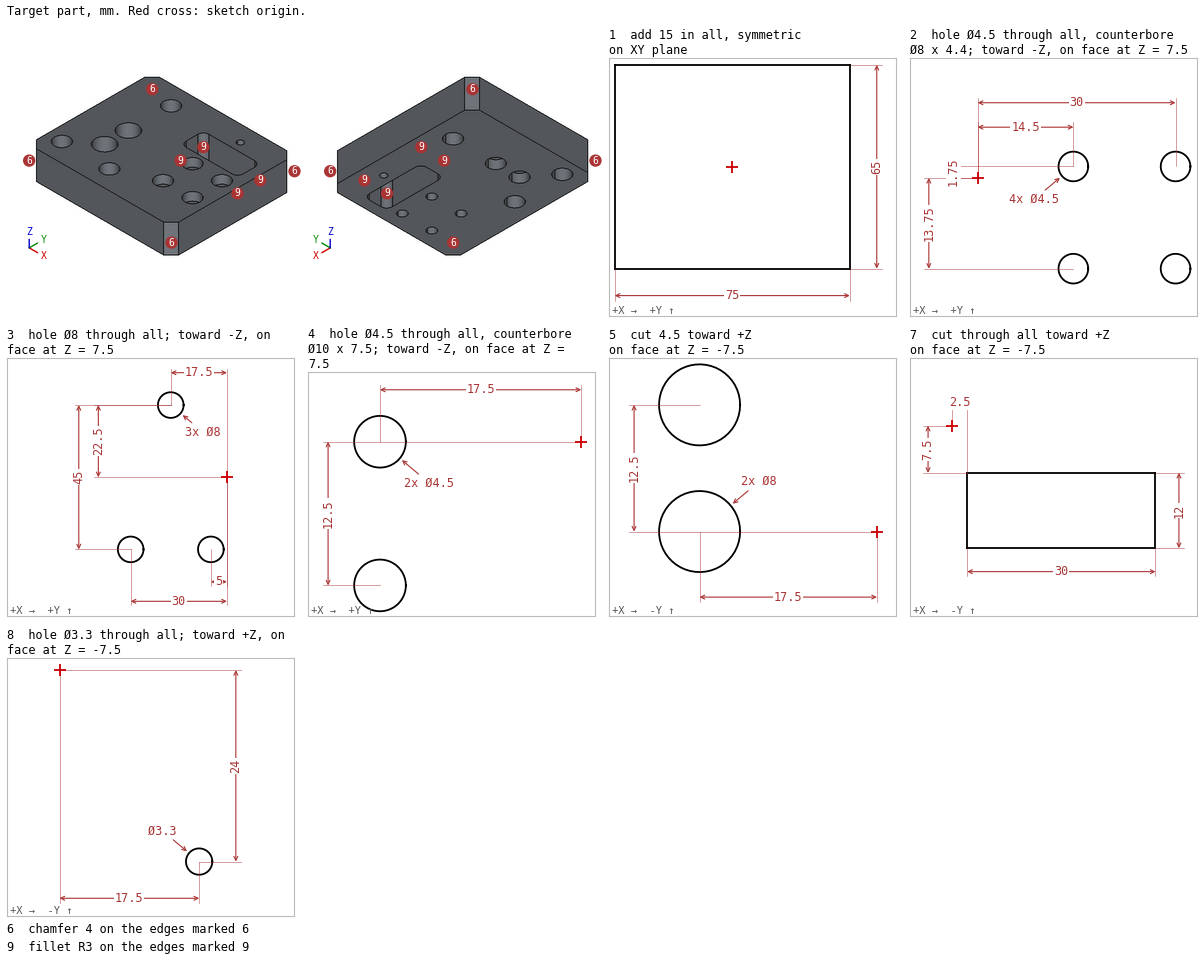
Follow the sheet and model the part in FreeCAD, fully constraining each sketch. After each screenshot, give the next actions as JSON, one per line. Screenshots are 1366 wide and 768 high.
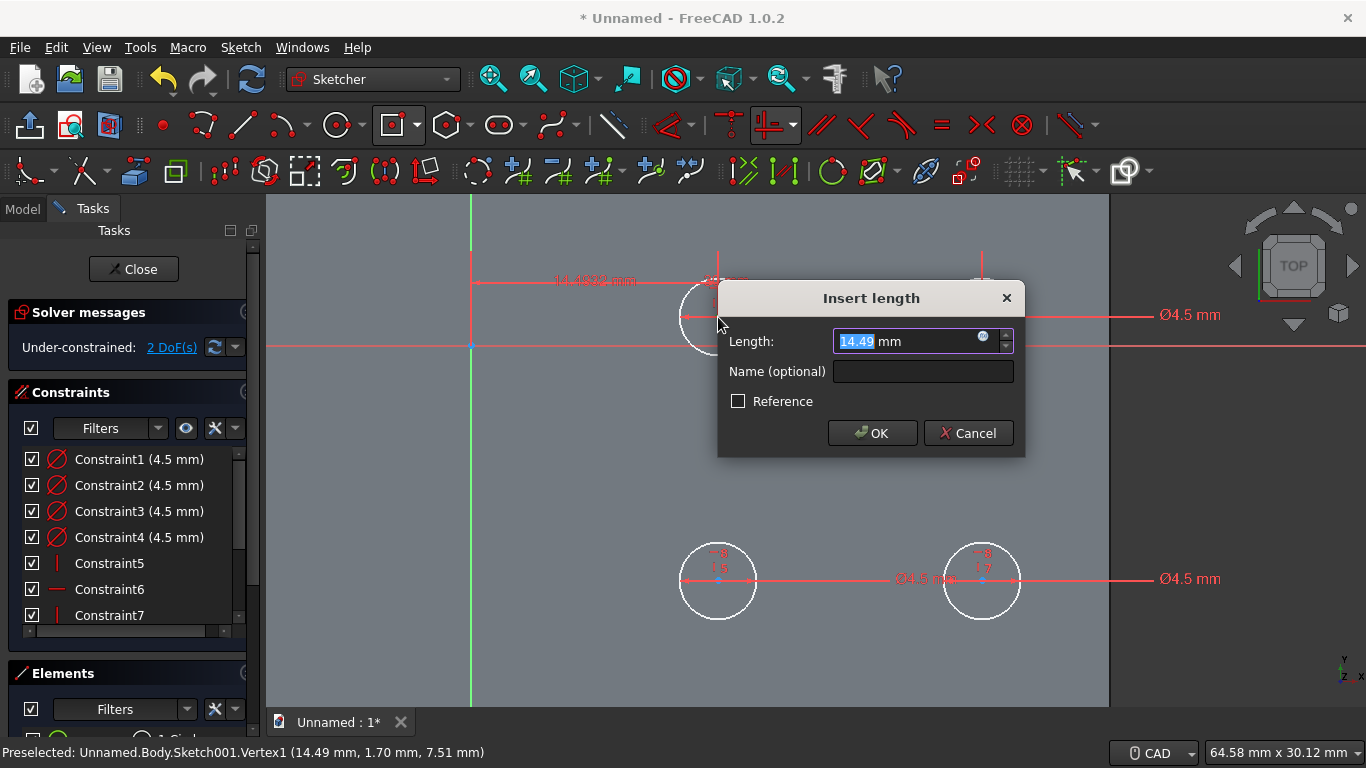
{"action": "type", "text": "14.5"}
{"action": "key", "text": "Return"}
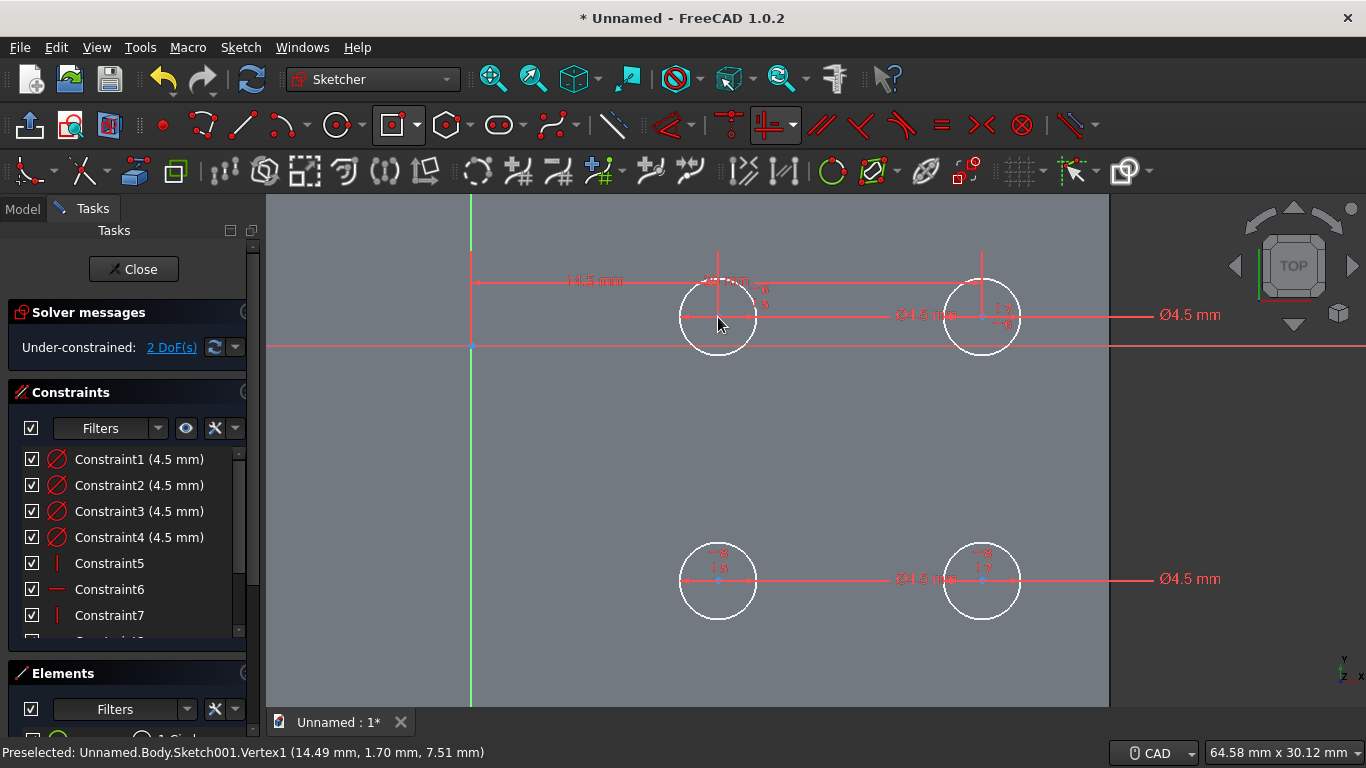
{"action": "scroll", "coordinate": [718, 317], "scroll_direction": "up", "scroll_amount": 2}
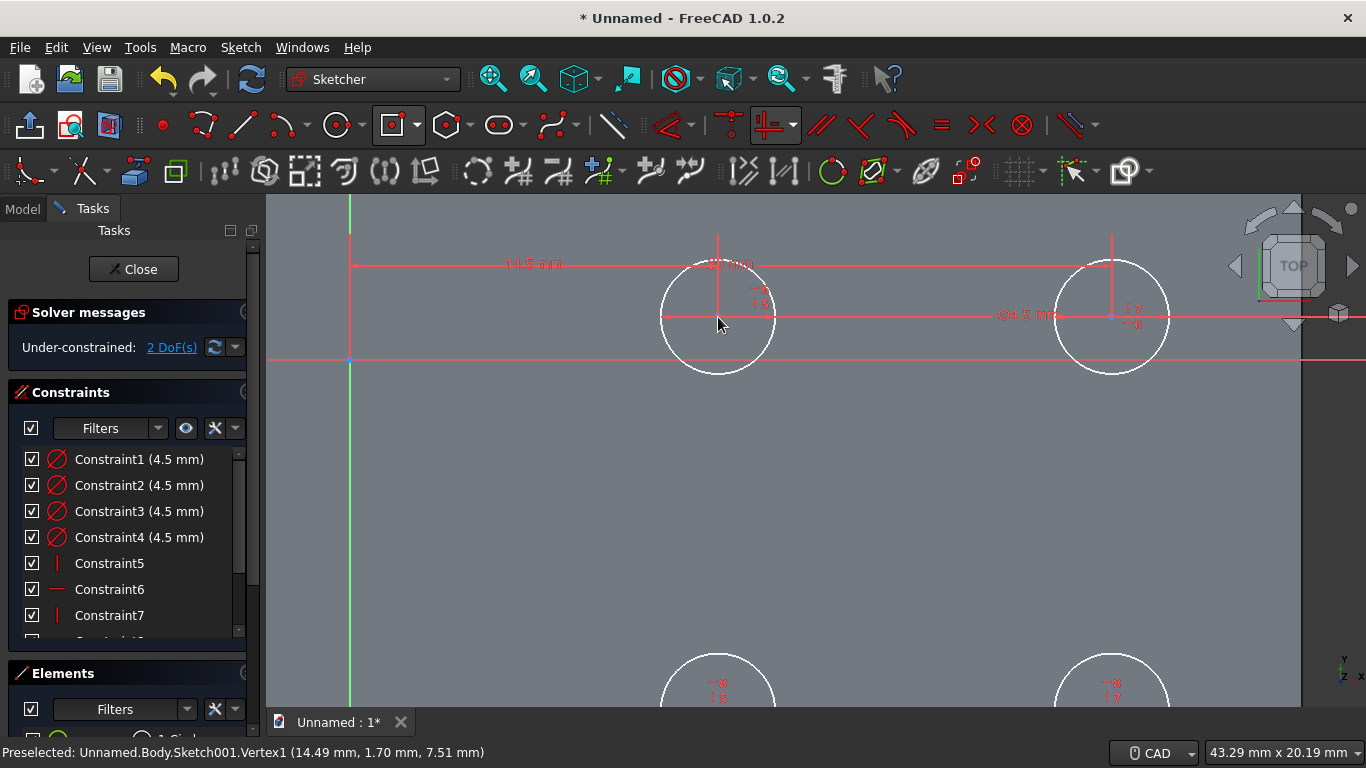
{"action": "left_click", "coordinate": [718, 317]}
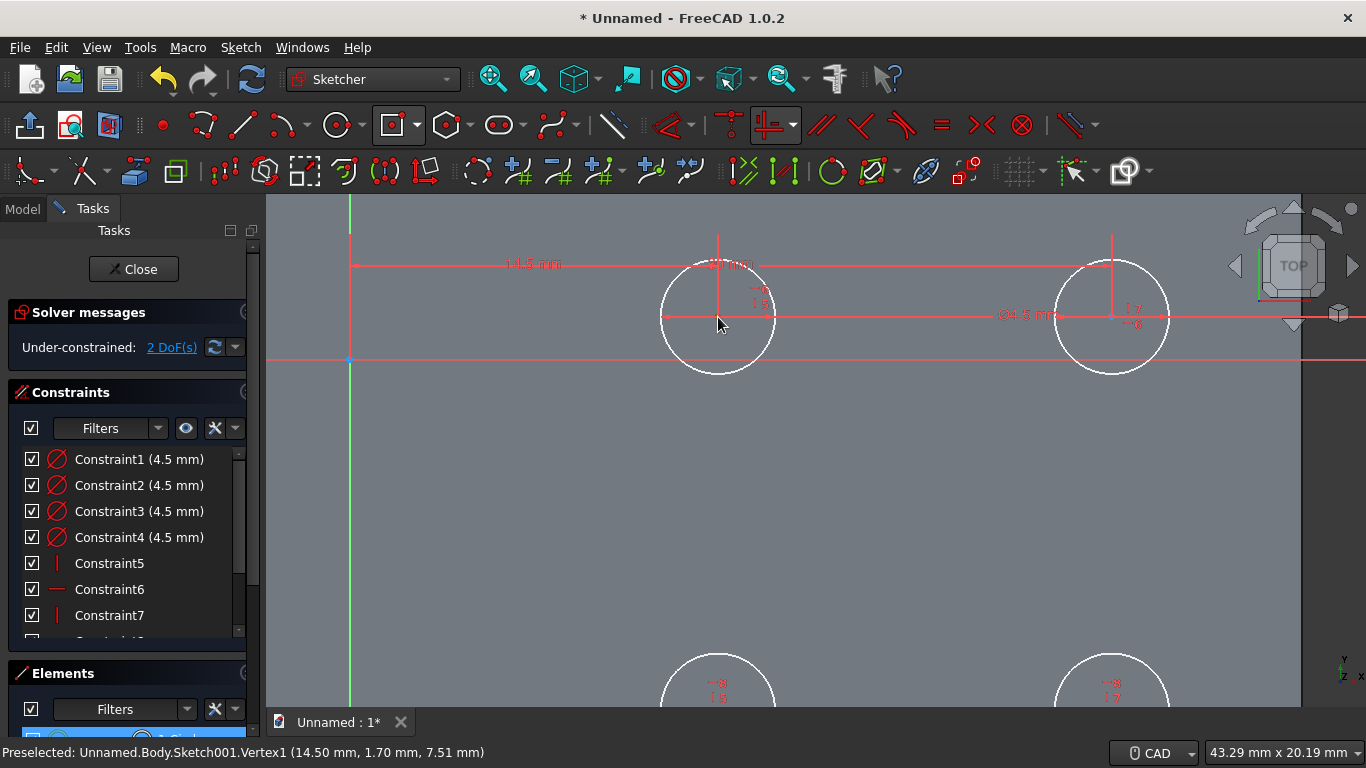
{"action": "key", "text": "i"}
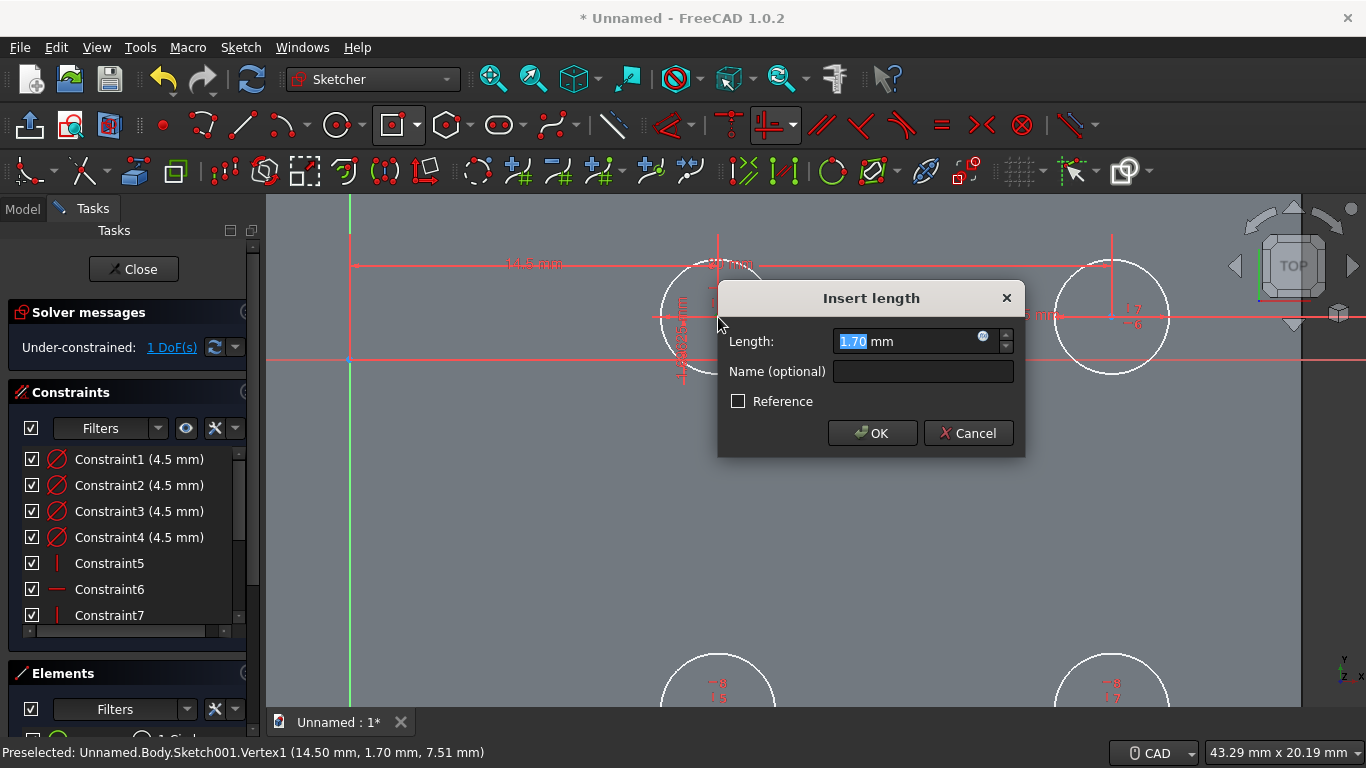
{"action": "type", "text": "1.75"}
{"action": "key", "text": "Return"}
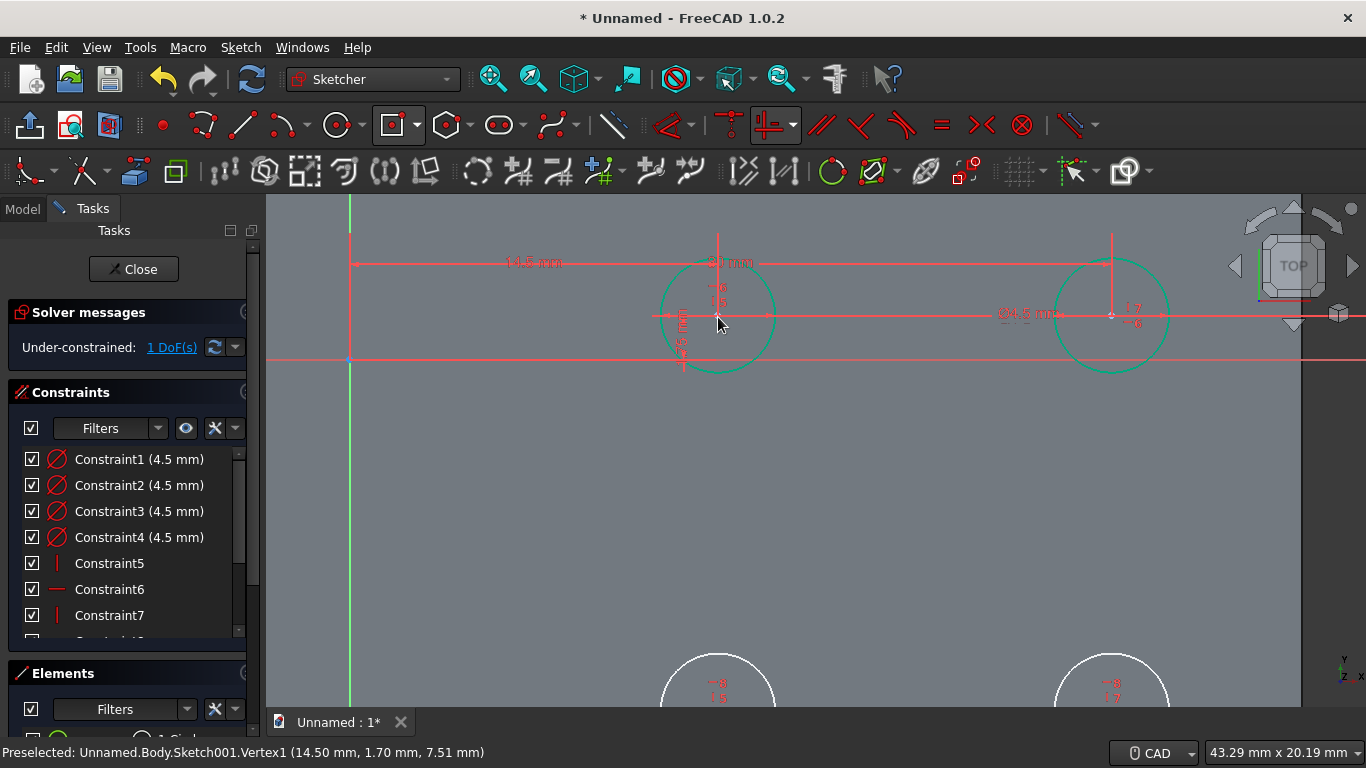
{"action": "scroll", "coordinate": [724, 325], "scroll_direction": "down", "scroll_amount": 2}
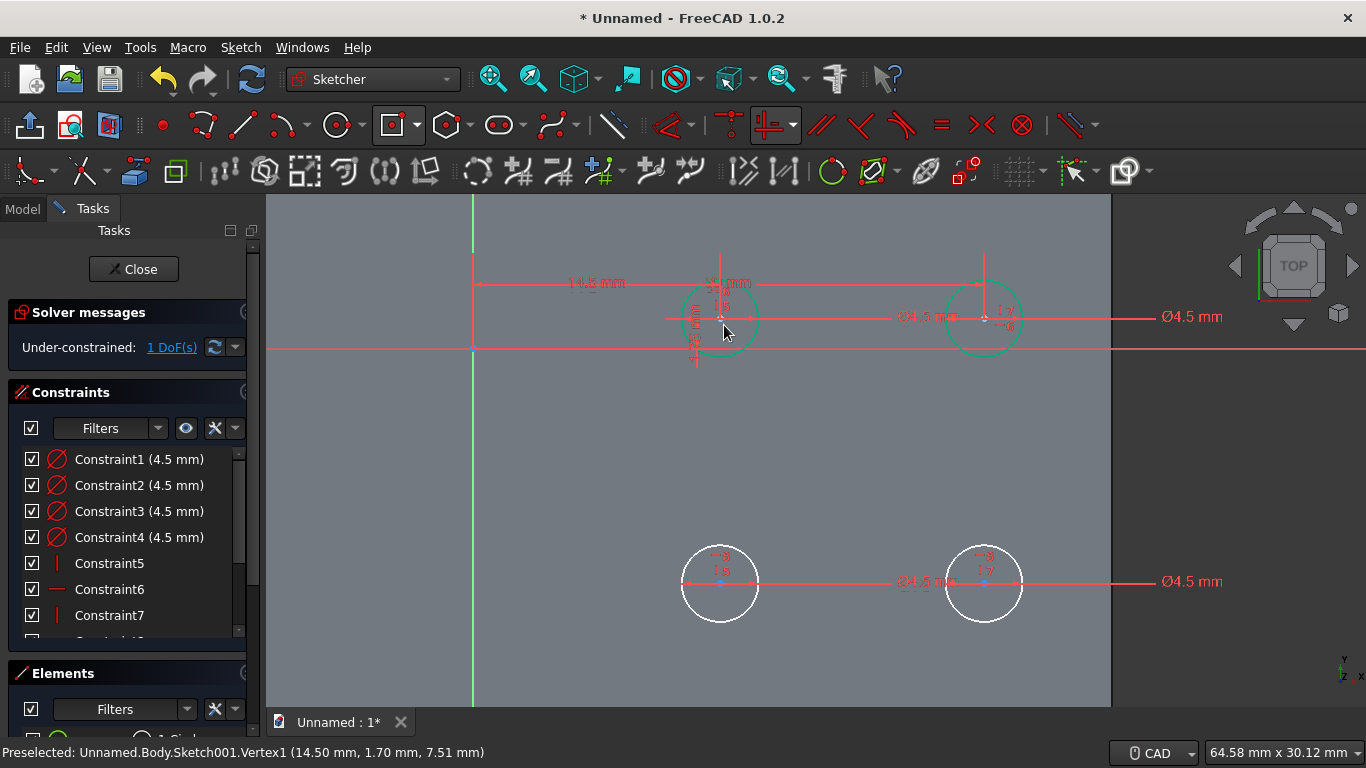
{"action": "left_click", "coordinate": [720, 584]}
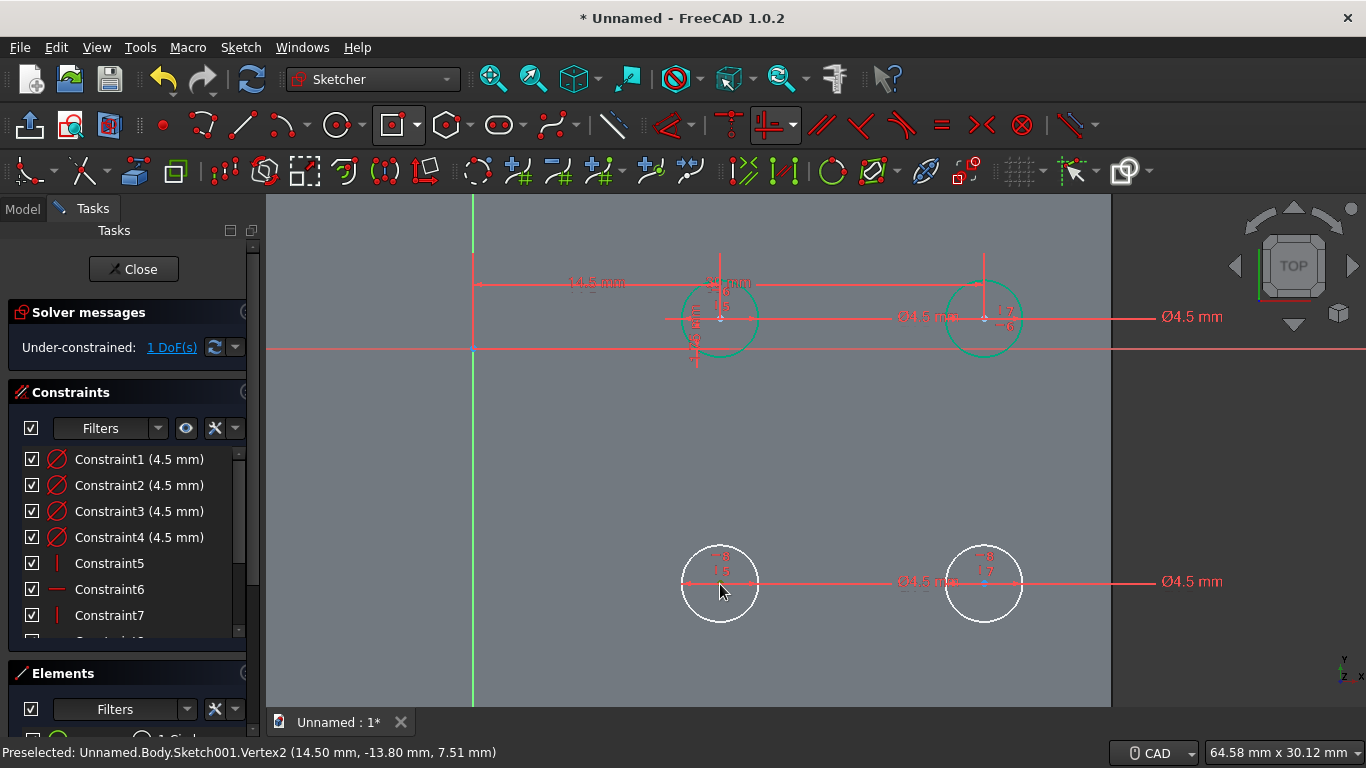
{"action": "key", "text": "i"}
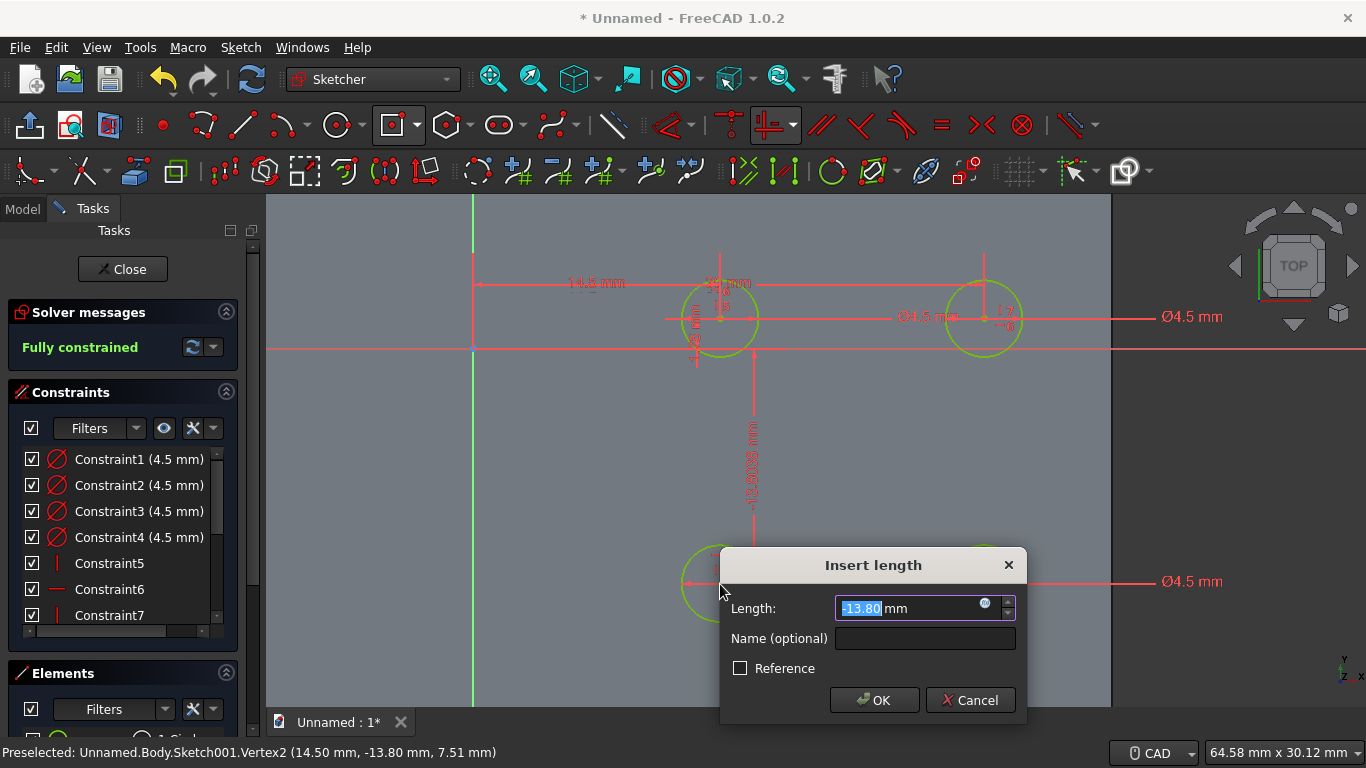
{"action": "type", "text": "-13.75"}
{"action": "key", "text": "Return"}